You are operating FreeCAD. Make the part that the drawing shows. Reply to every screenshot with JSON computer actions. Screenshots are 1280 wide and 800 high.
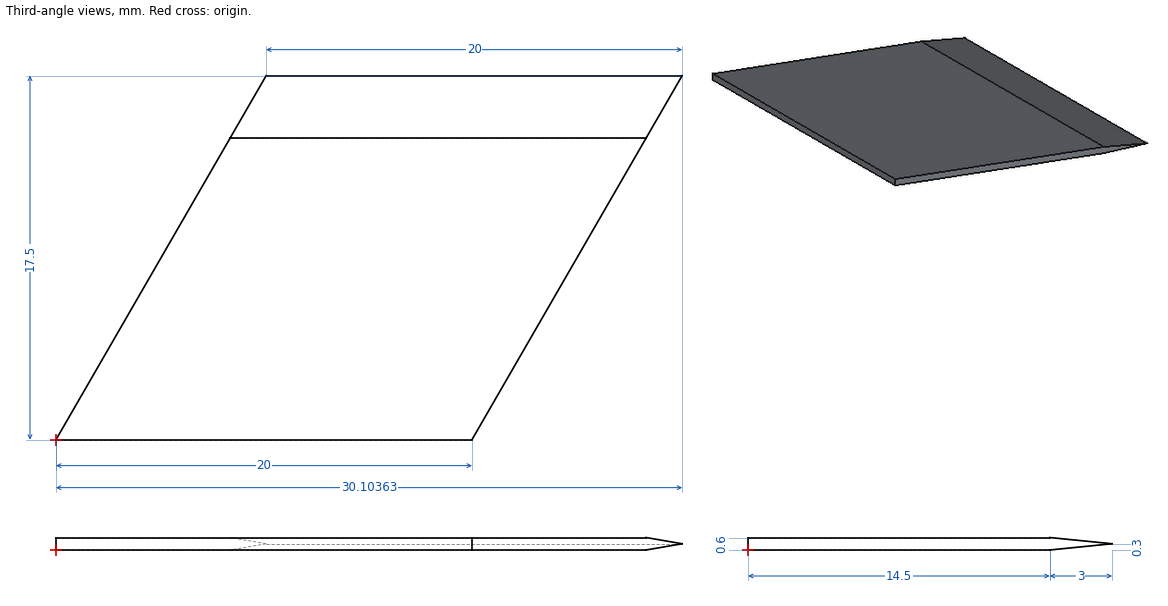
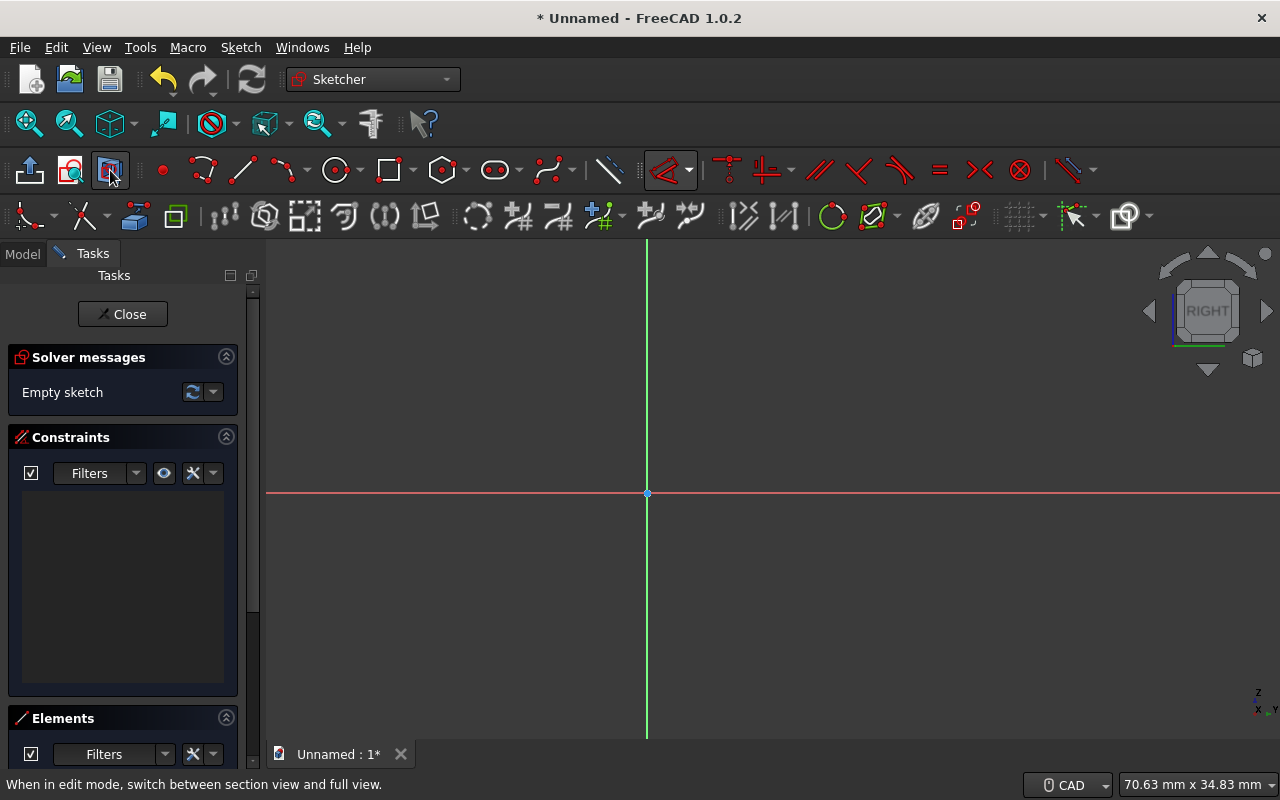
{"action": "scroll", "coordinate": [891, 491], "scroll_direction": "up", "scroll_amount": 13}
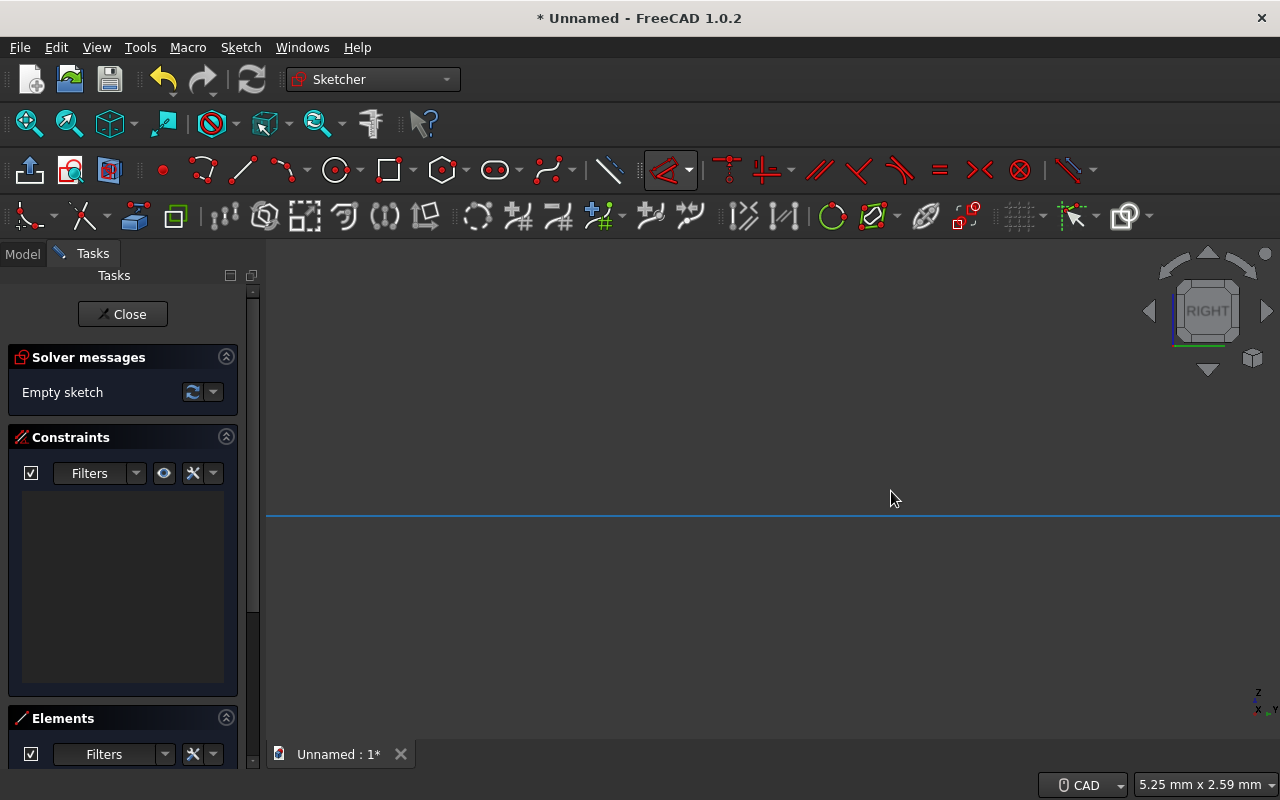
{"action": "left_click", "coordinate": [204, 170]}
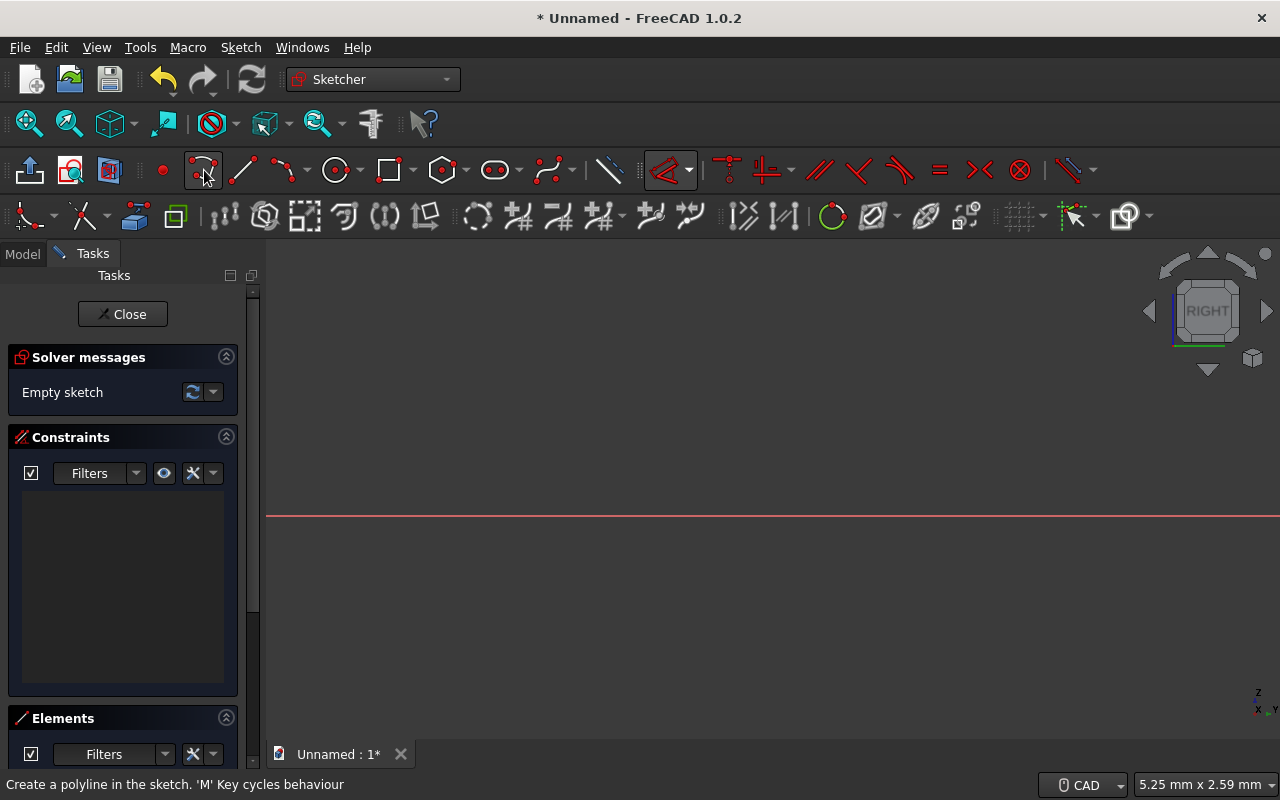
{"action": "left_click", "coordinate": [406, 516]}
{"action": "left_click", "coordinate": [986, 507]}
{"action": "left_click", "coordinate": [986, 458]}
{"action": "left_click", "coordinate": [406, 516]}
{"action": "key", "text": "Escape"}
{"action": "key", "text": "Escape"}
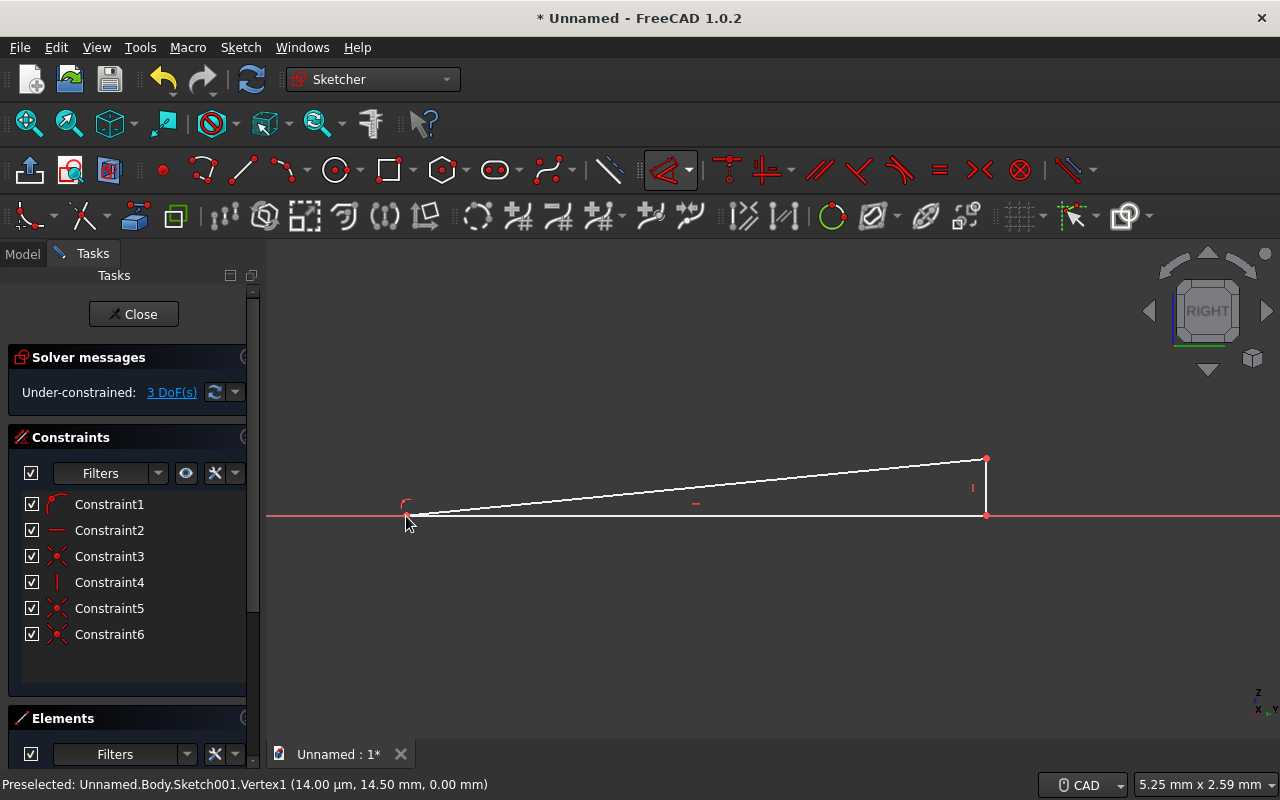
{"action": "left_click", "coordinate": [580, 516]}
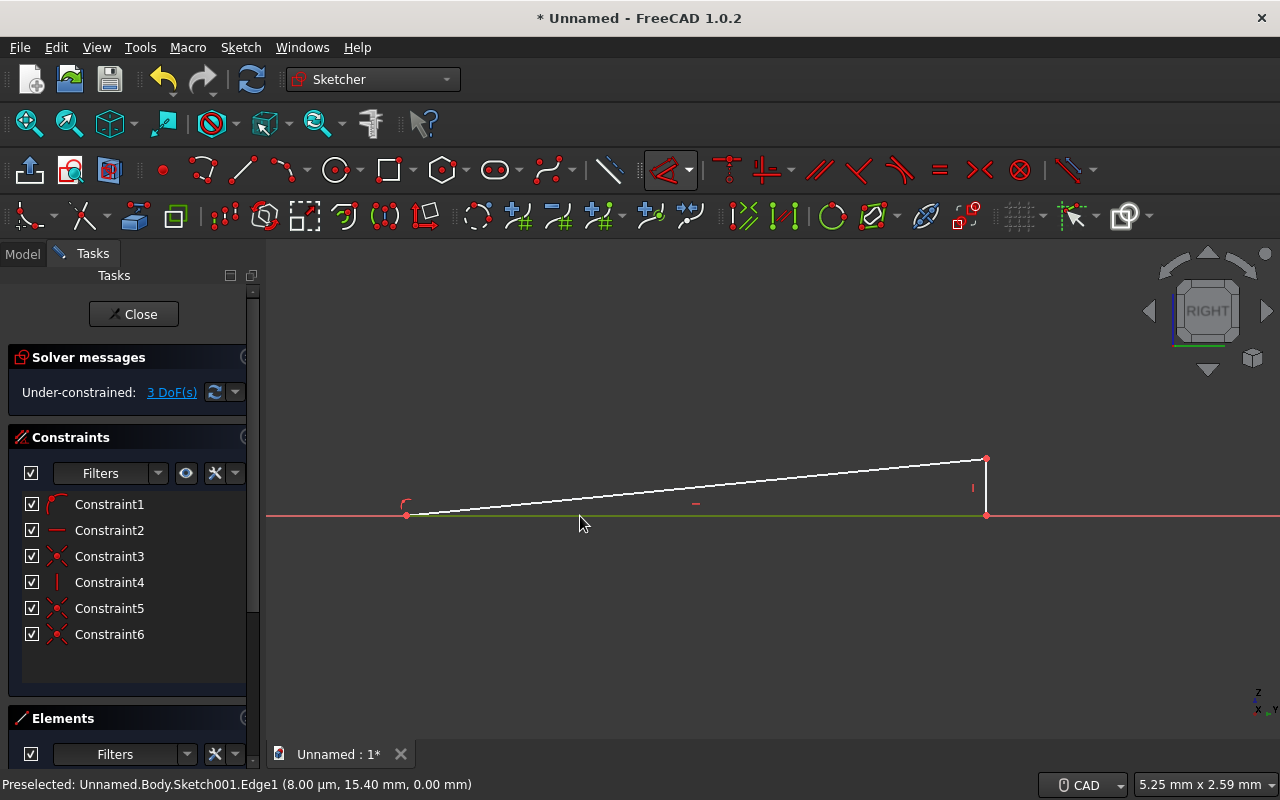
{"action": "key", "text": "l"}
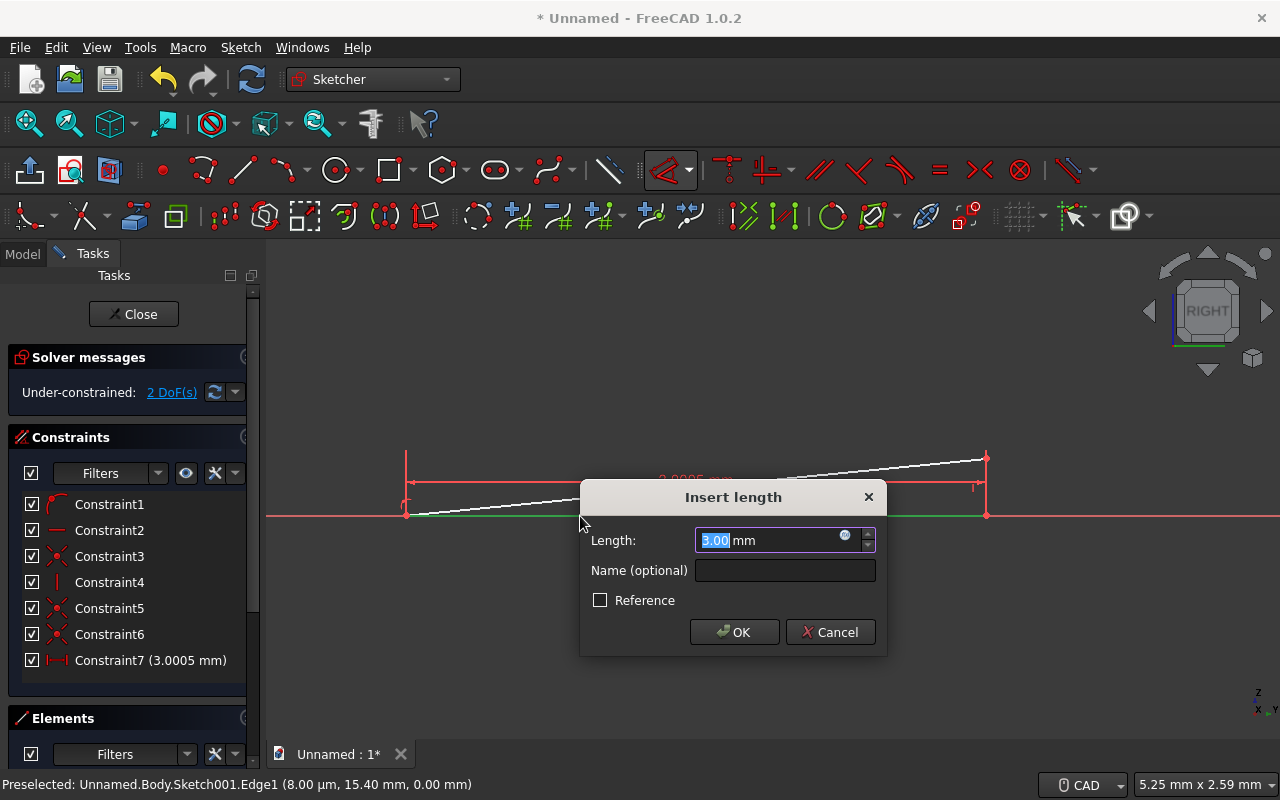
{"action": "type", "text": "3"}
{"action": "key", "text": "Return"}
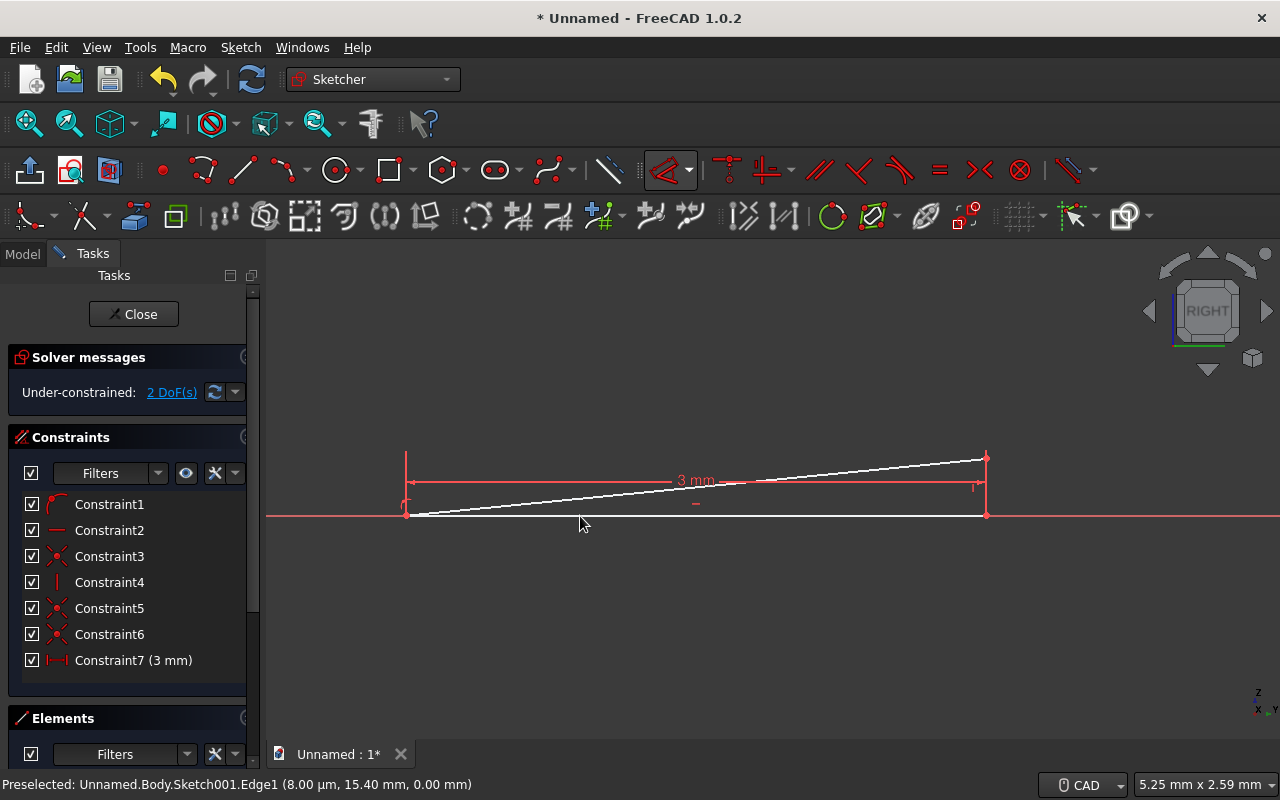
{"action": "left_click", "coordinate": [986, 499]}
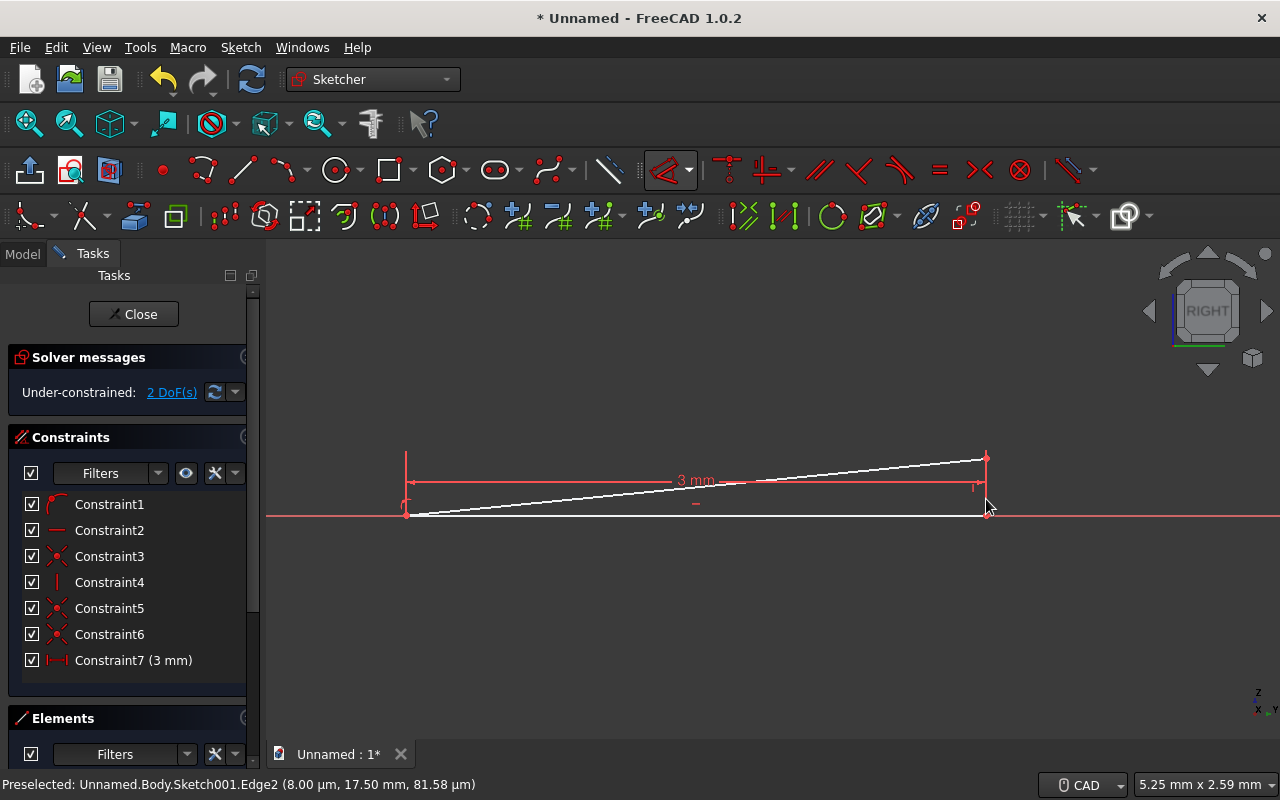
{"action": "left_click", "coordinate": [692, 170]}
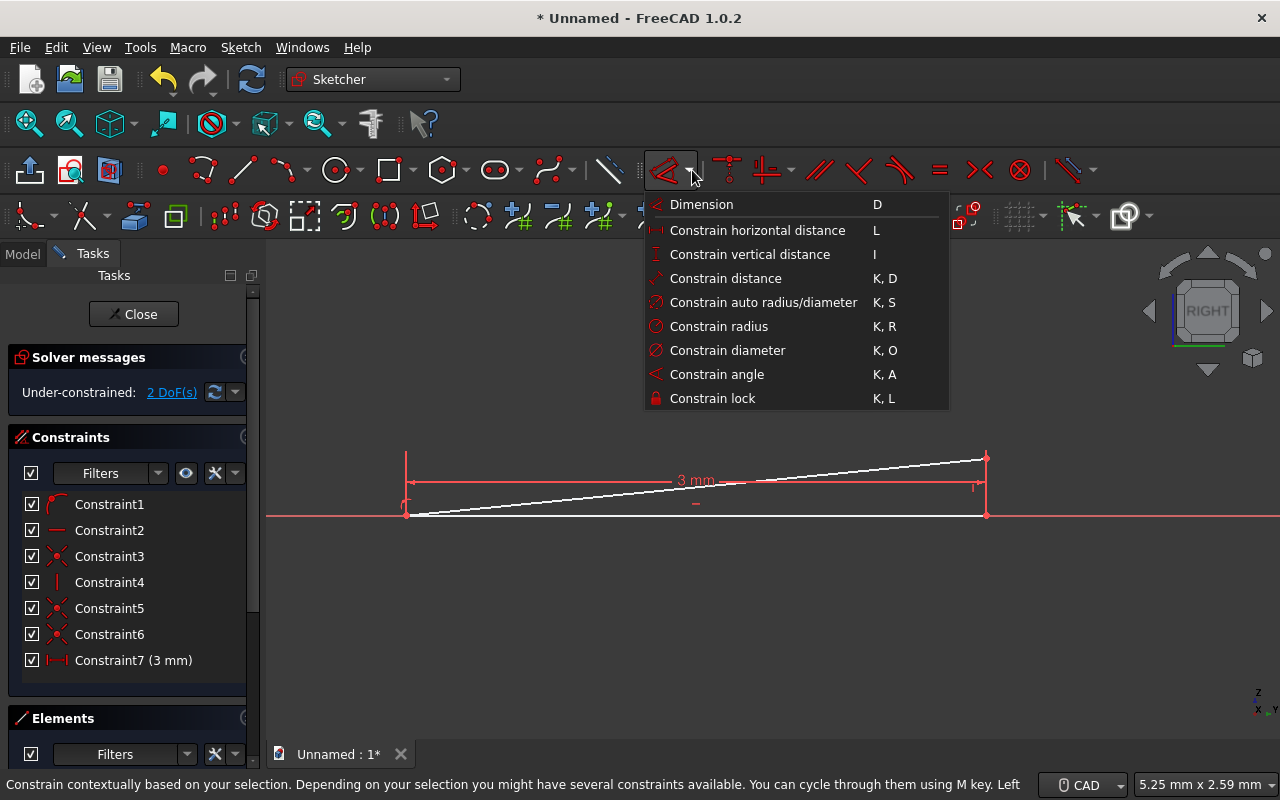
{"action": "left_click", "coordinate": [797, 254]}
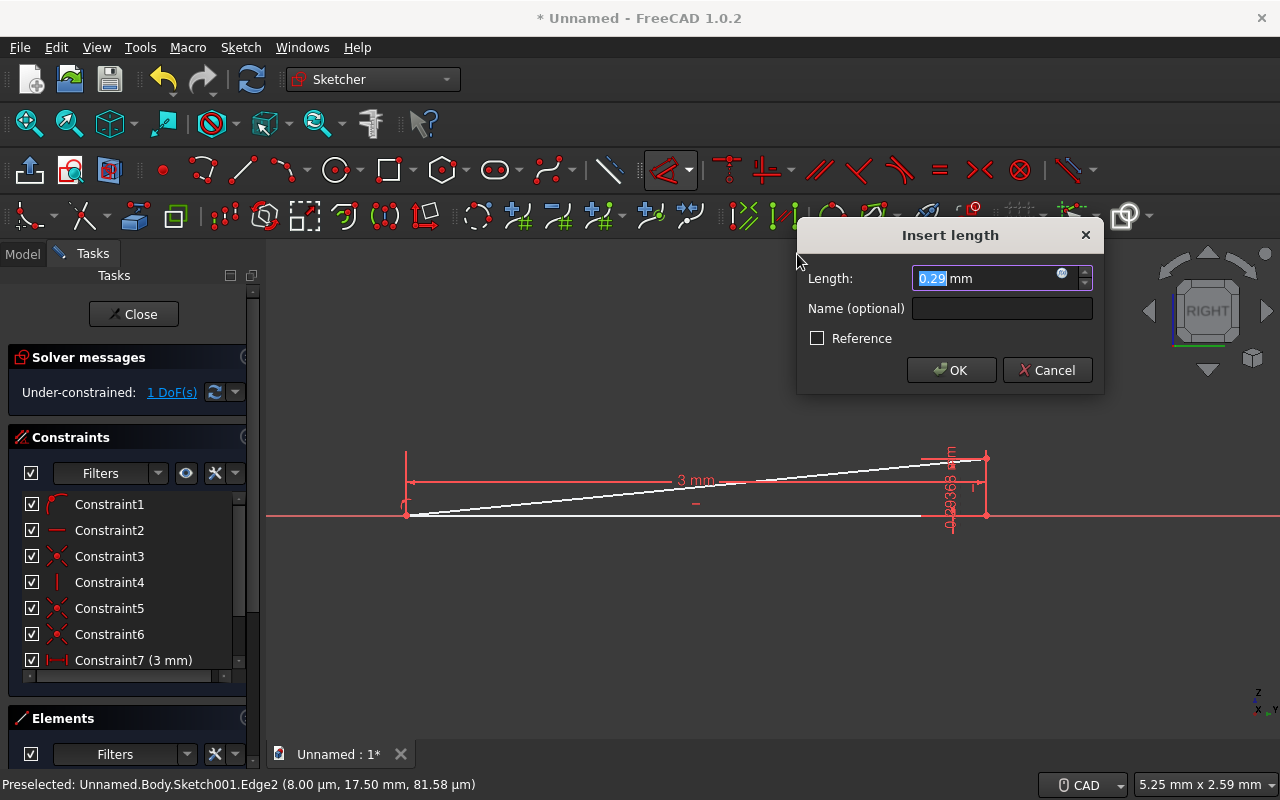
{"action": "type", "text": "0.3"}
{"action": "key", "text": "Return"}